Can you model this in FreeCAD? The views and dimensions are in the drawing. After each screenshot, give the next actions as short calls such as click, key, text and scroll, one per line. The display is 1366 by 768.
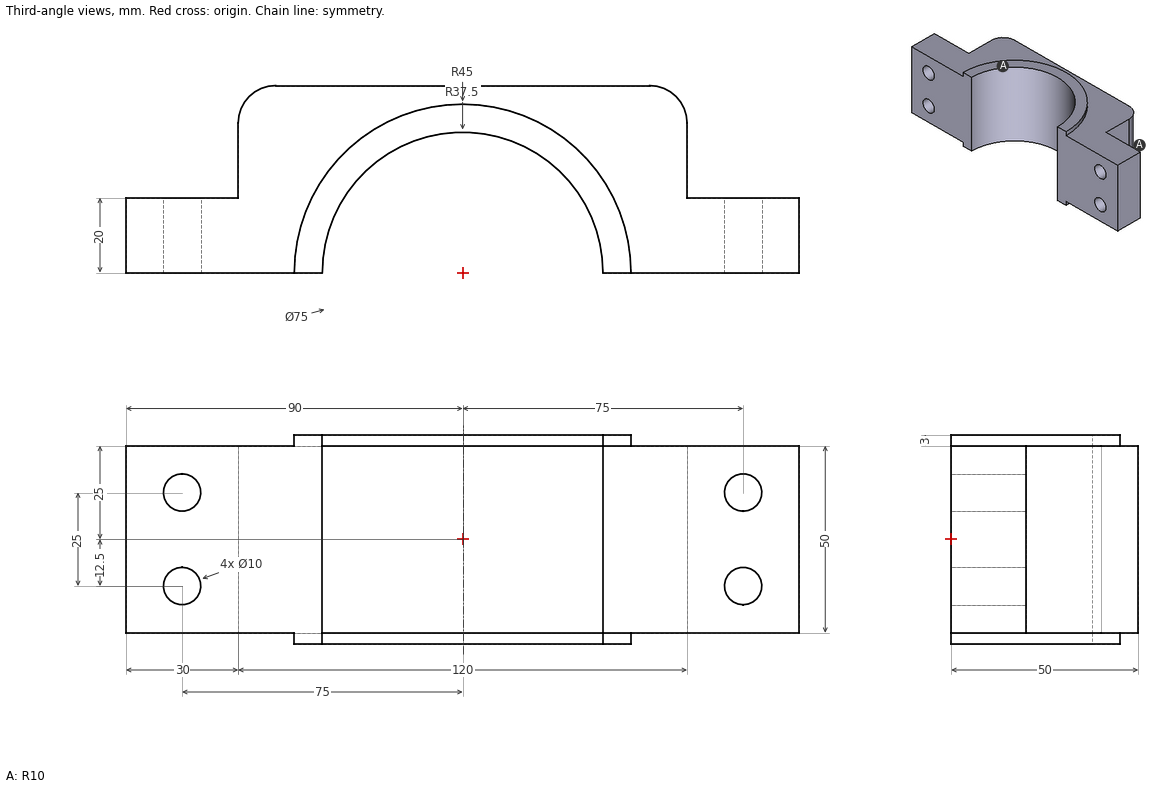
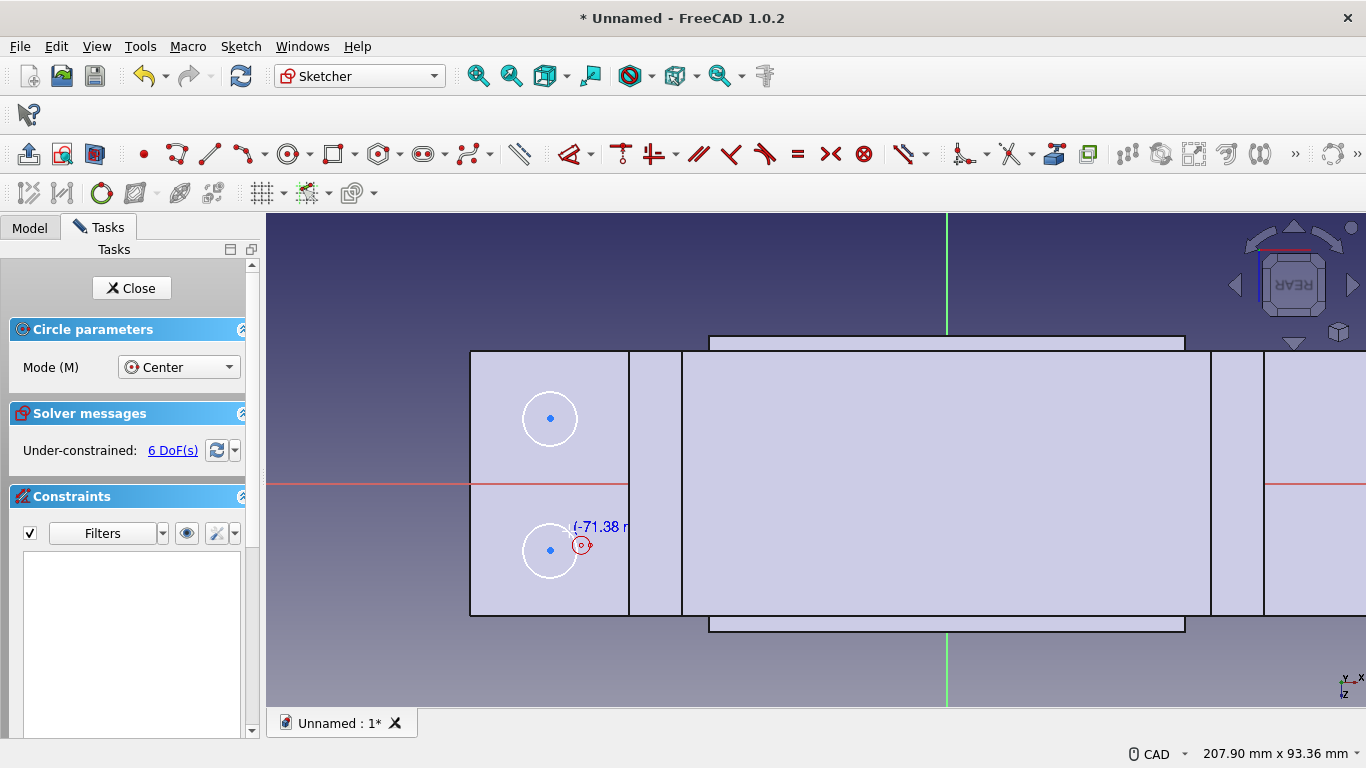
scroll(294, 353, down, 1)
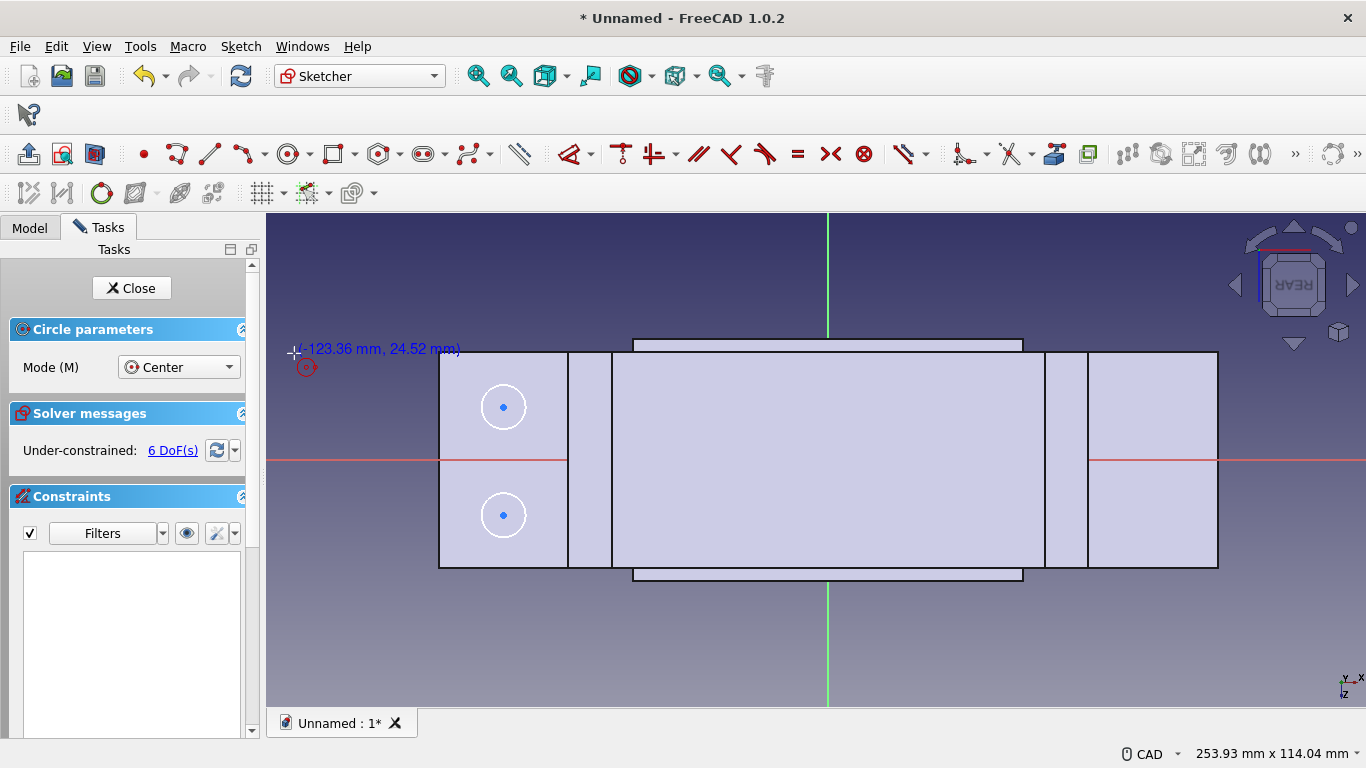
click(1153, 514)
click(1169, 499)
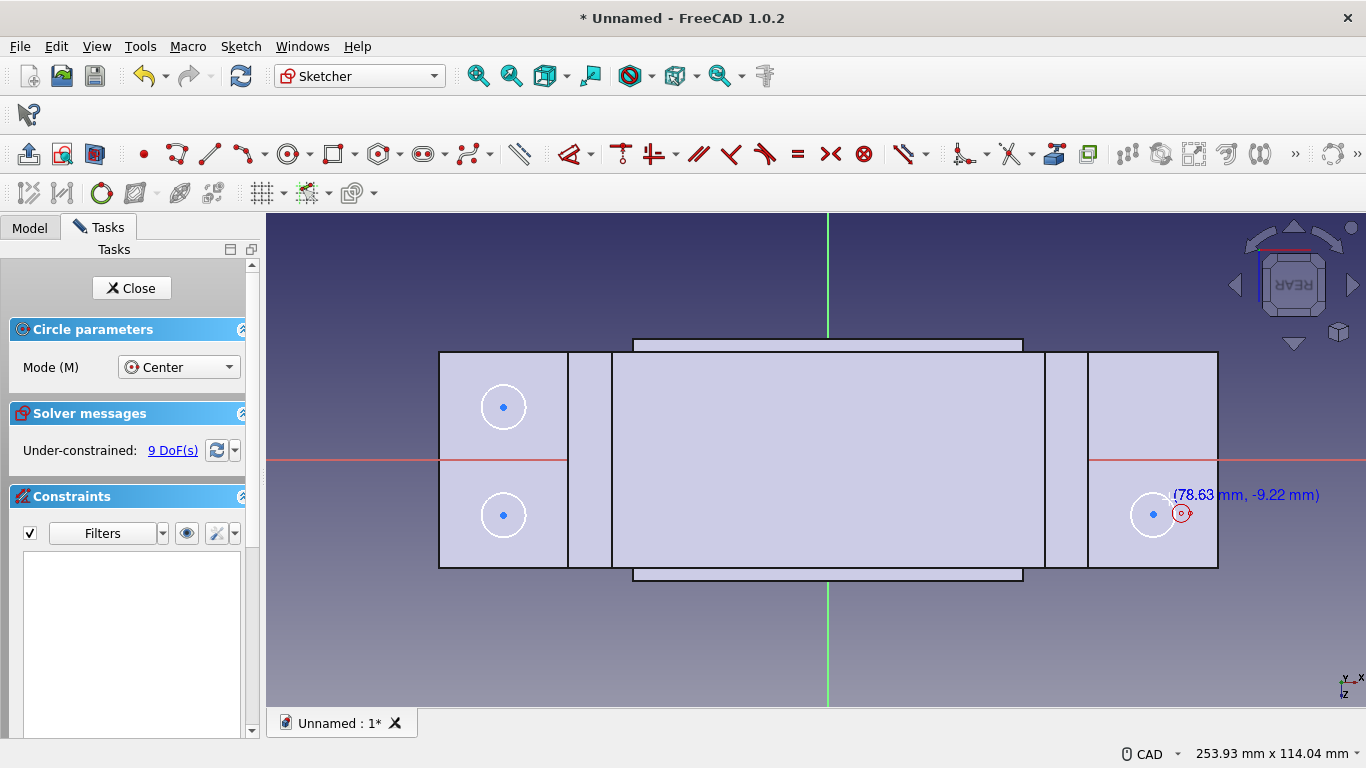
click(1153, 406)
click(1169, 391)
key(Escape)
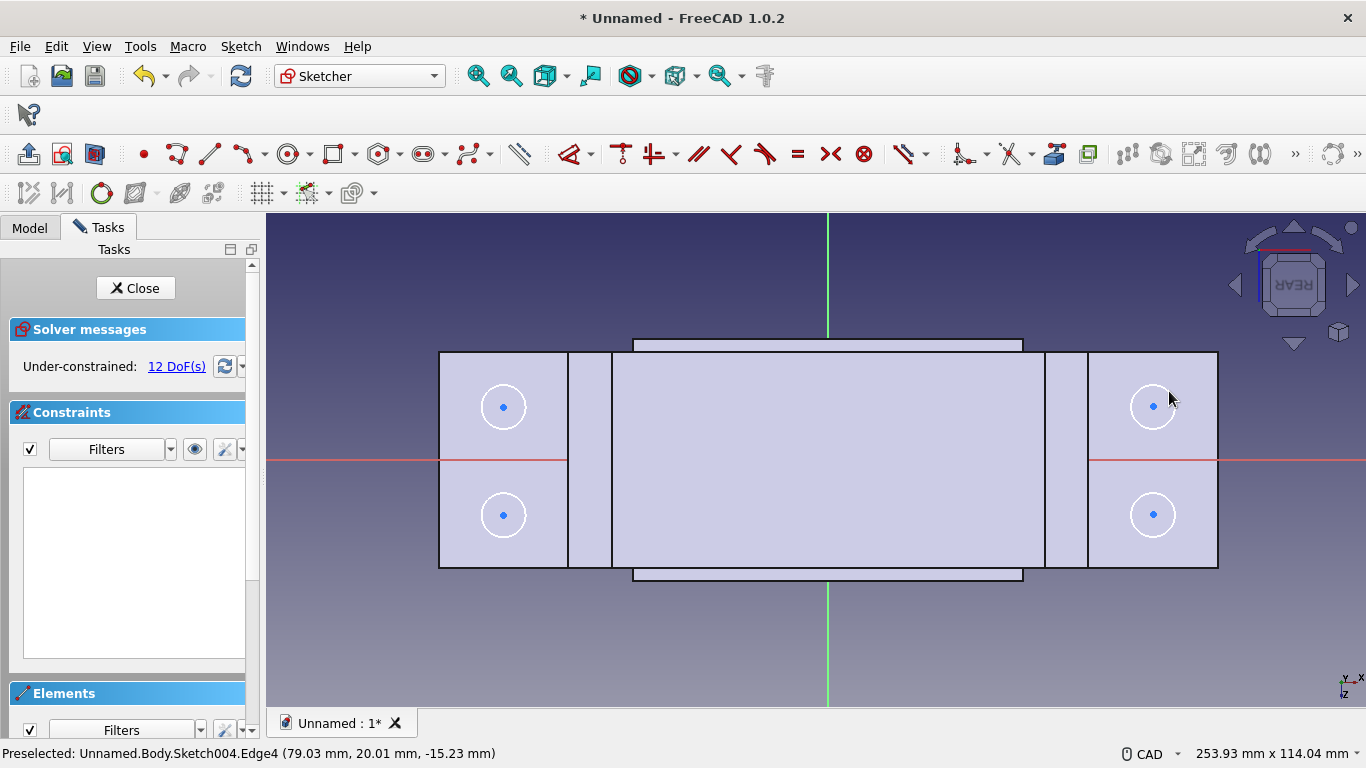
click(519, 391)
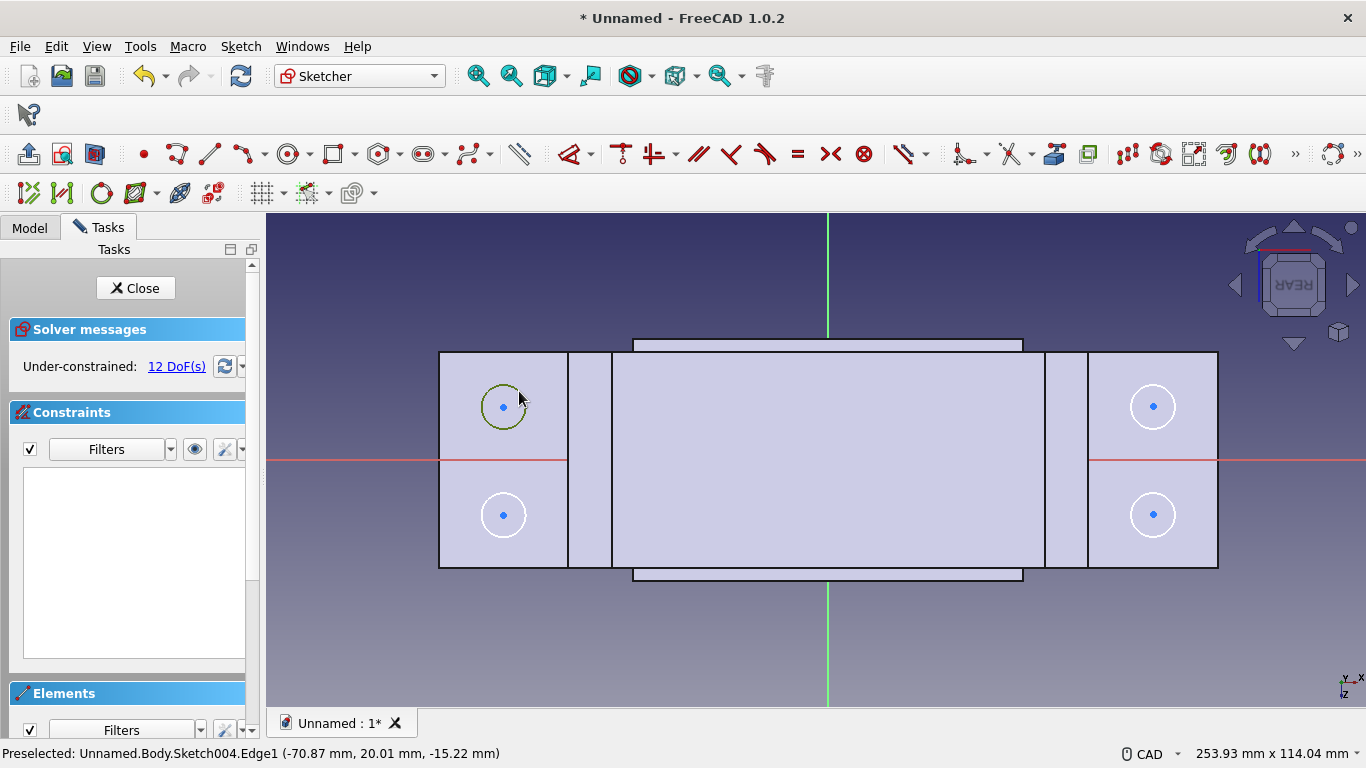
click(519, 500)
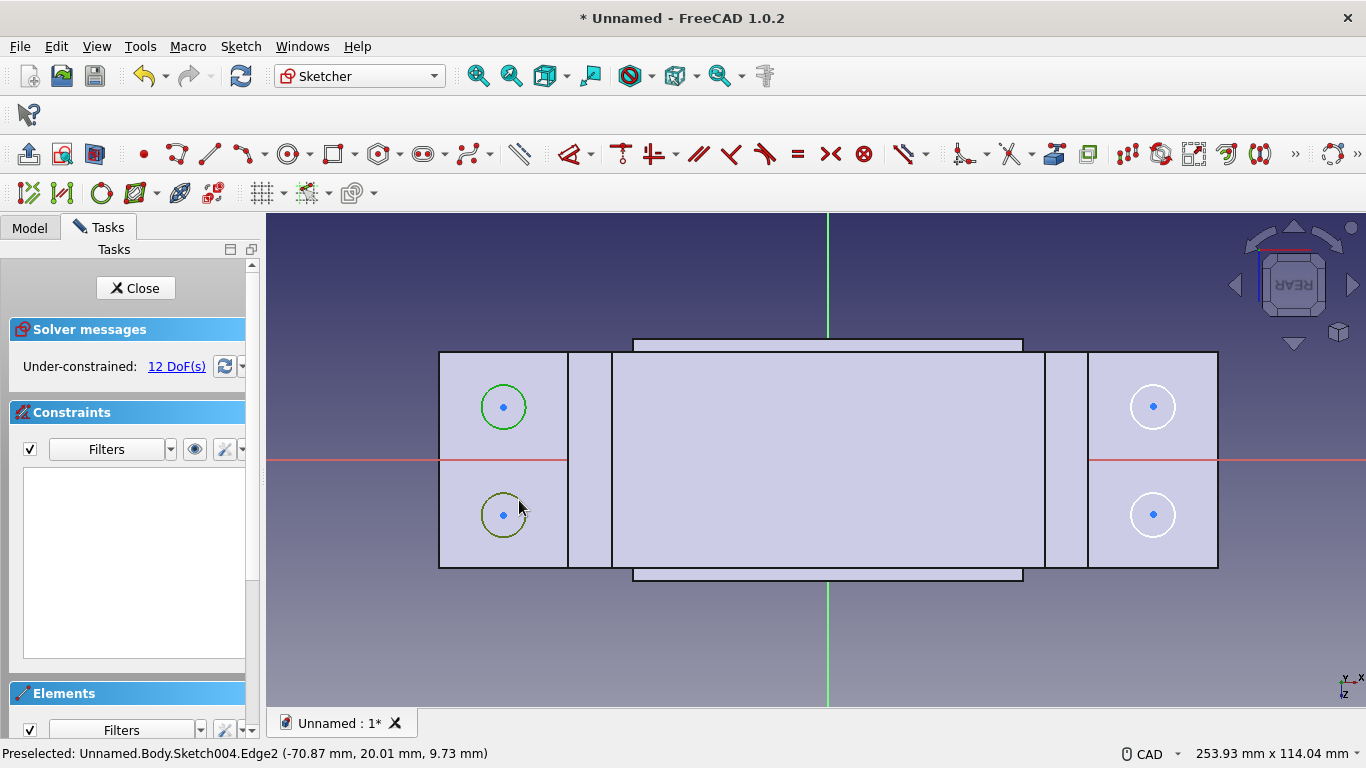
click(1168, 499)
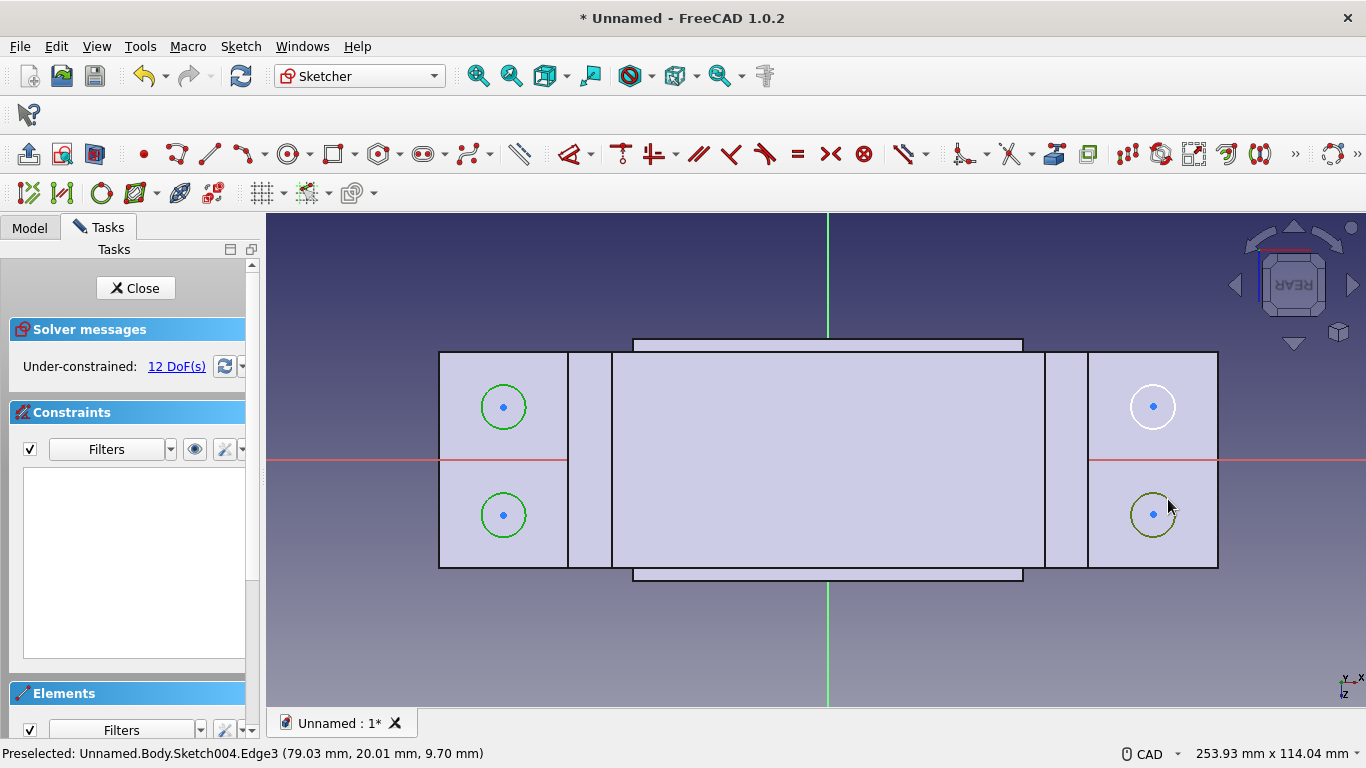
click(1168, 391)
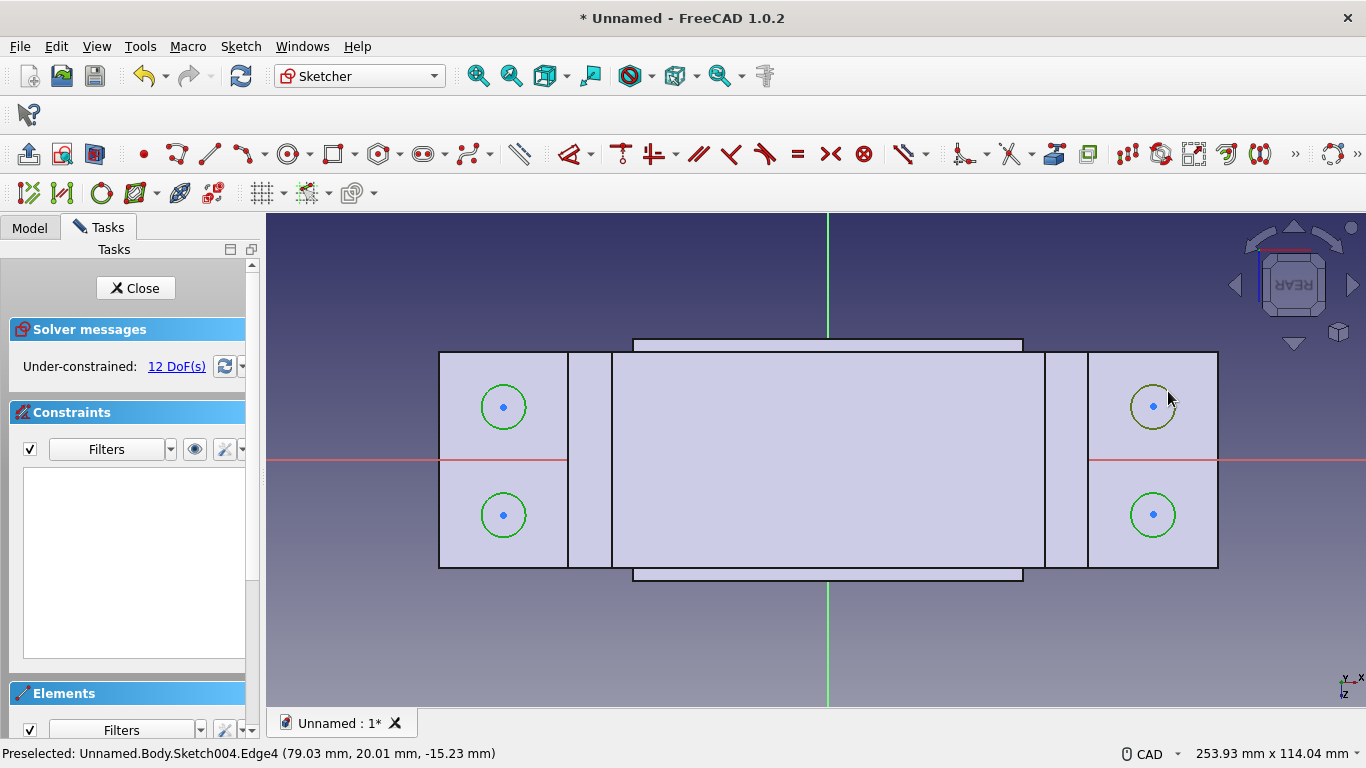
click(798, 154)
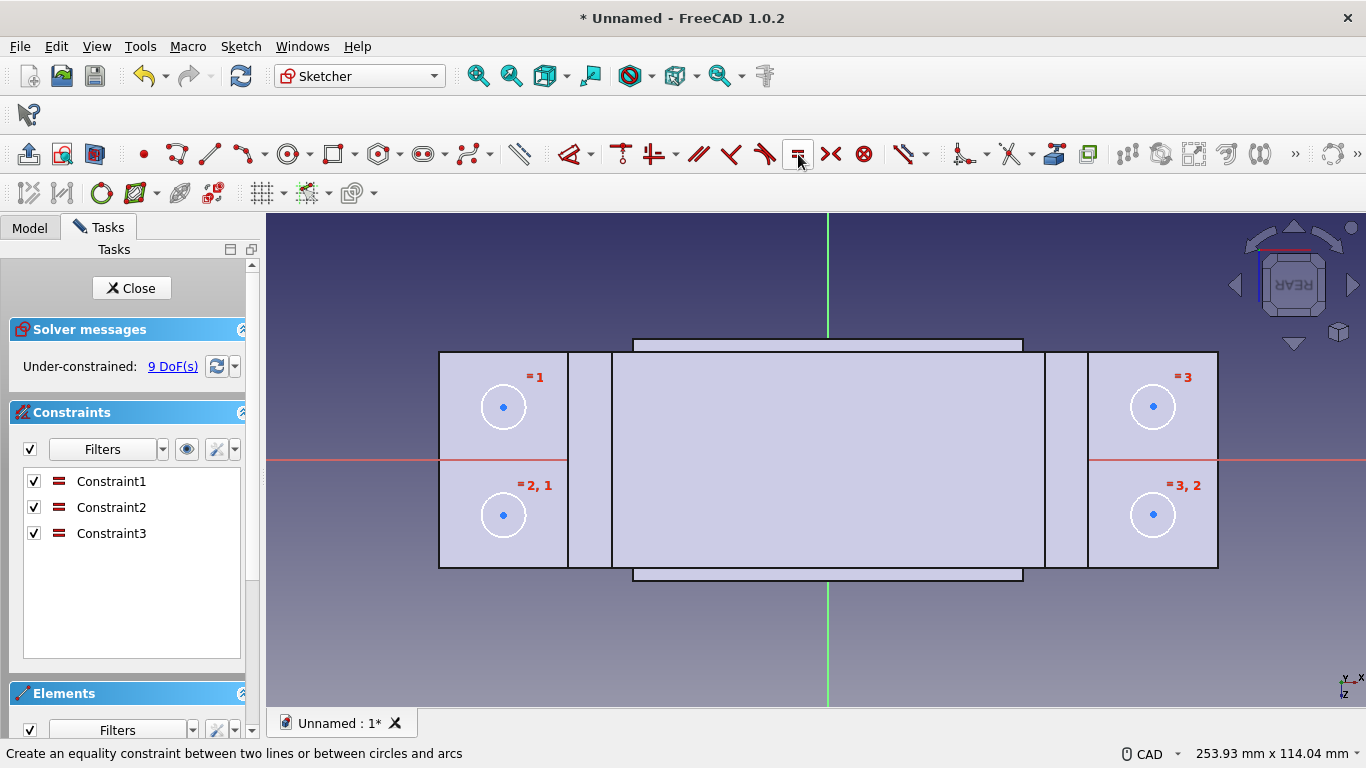
click(504, 407)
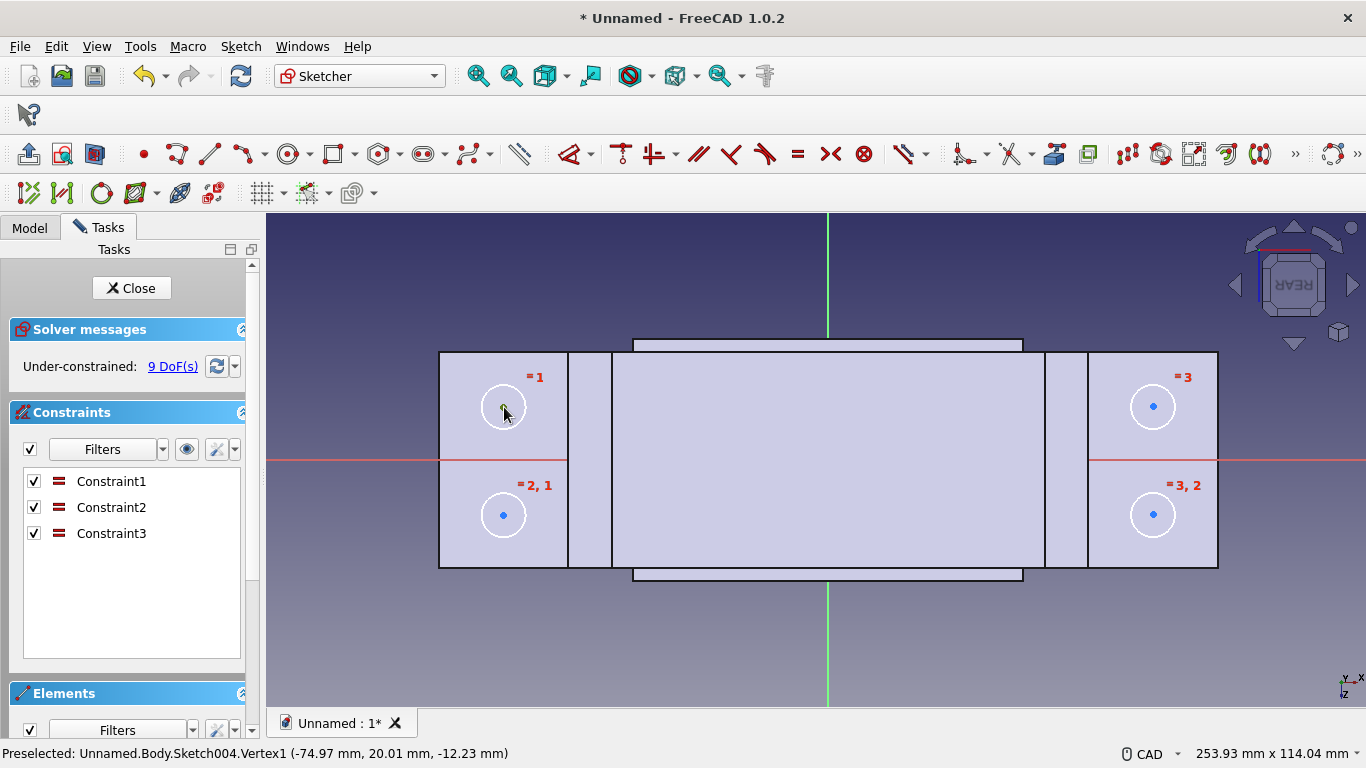
click(504, 515)